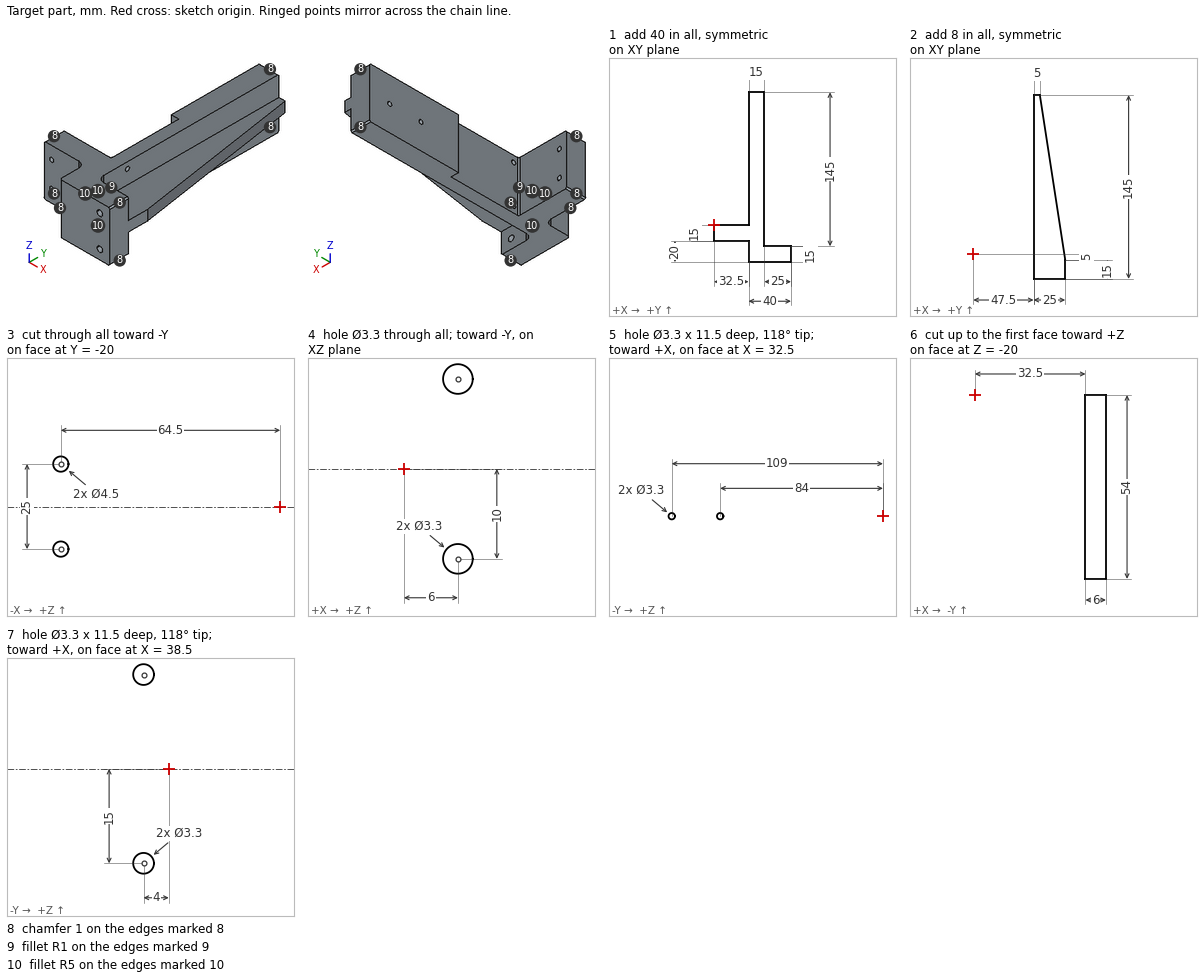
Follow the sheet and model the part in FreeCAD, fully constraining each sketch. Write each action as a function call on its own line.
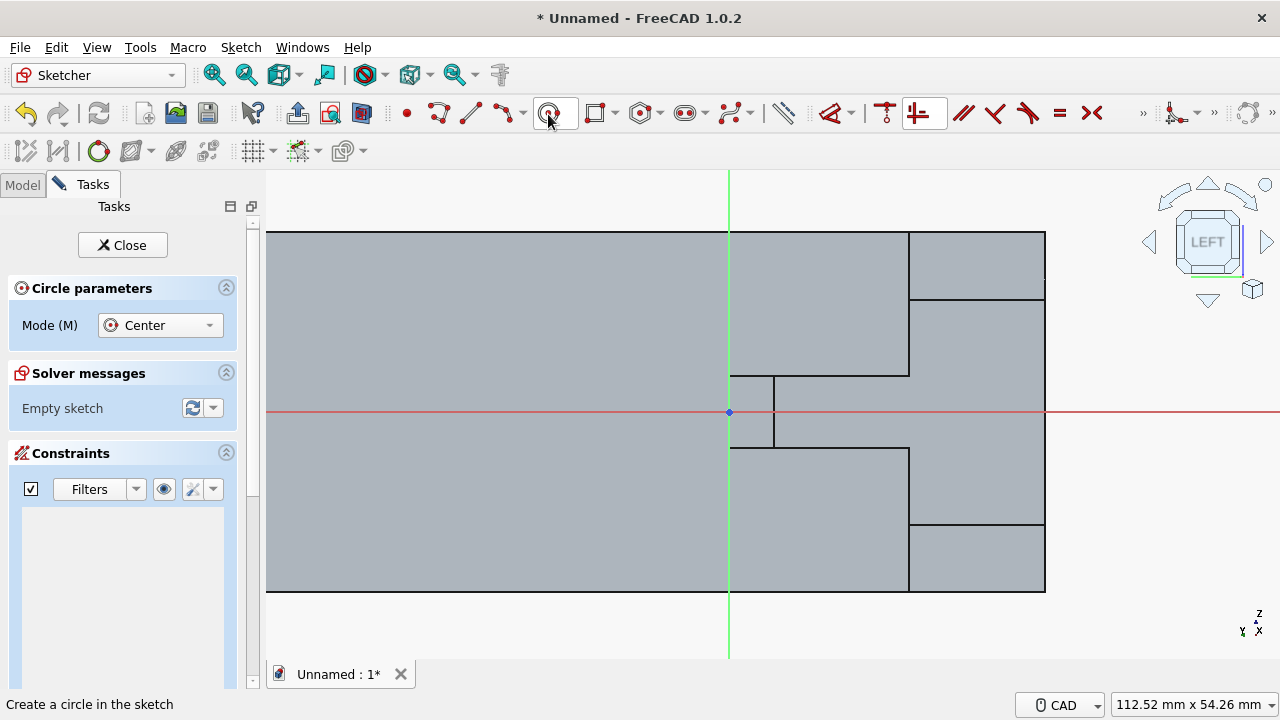
scroll(693, 547, up, 3)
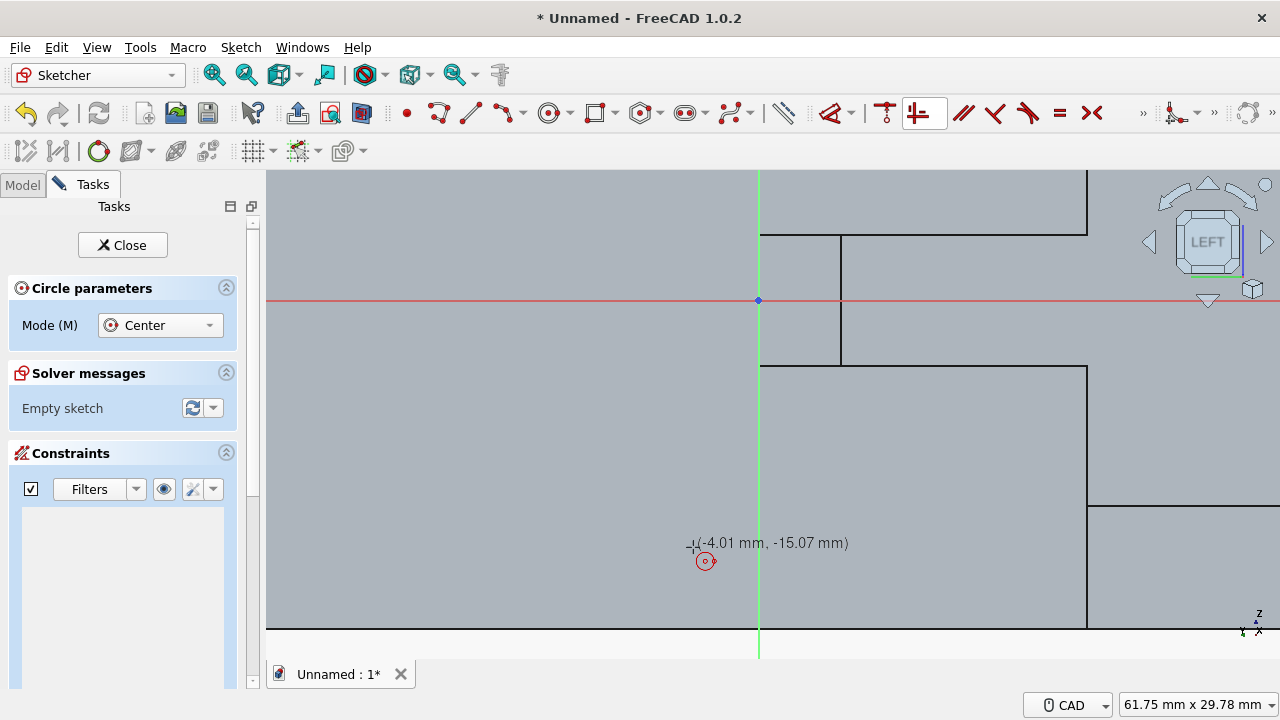
click(693, 547)
click(712, 528)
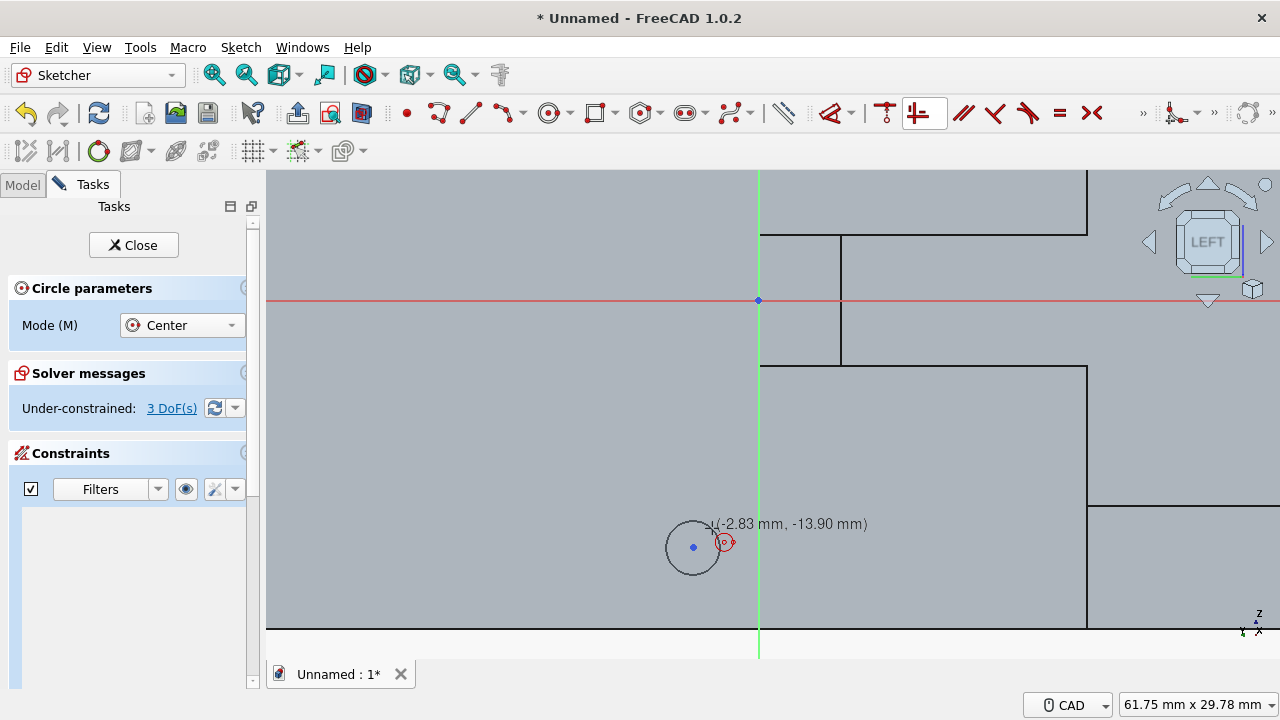
scroll(695, 553, down, 3)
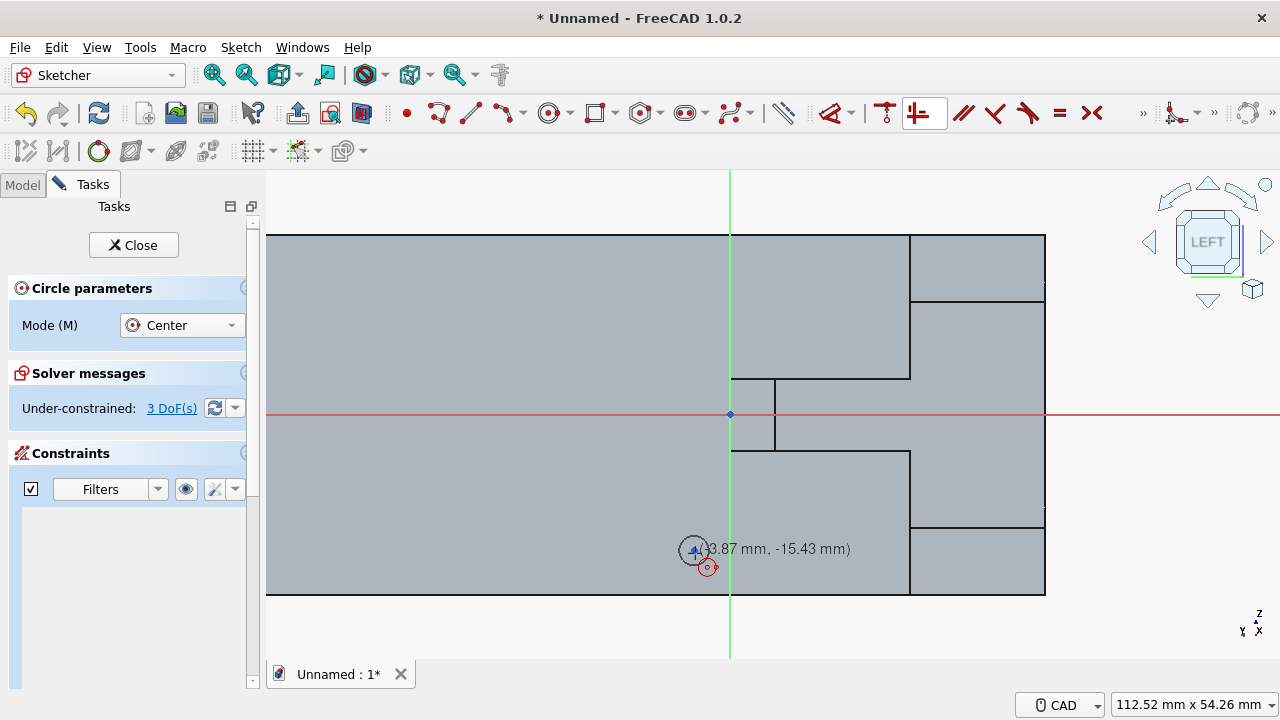
scroll(694, 280, up, 3)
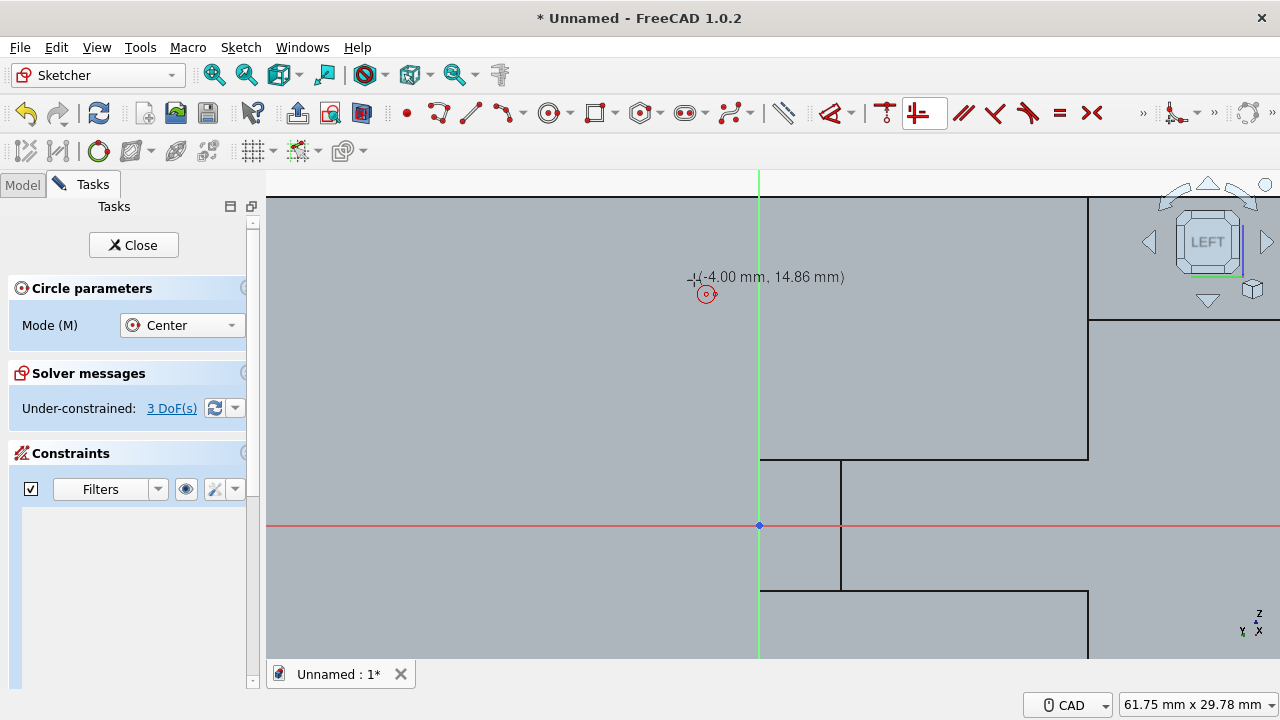
click(694, 279)
click(713, 260)
key(Escape)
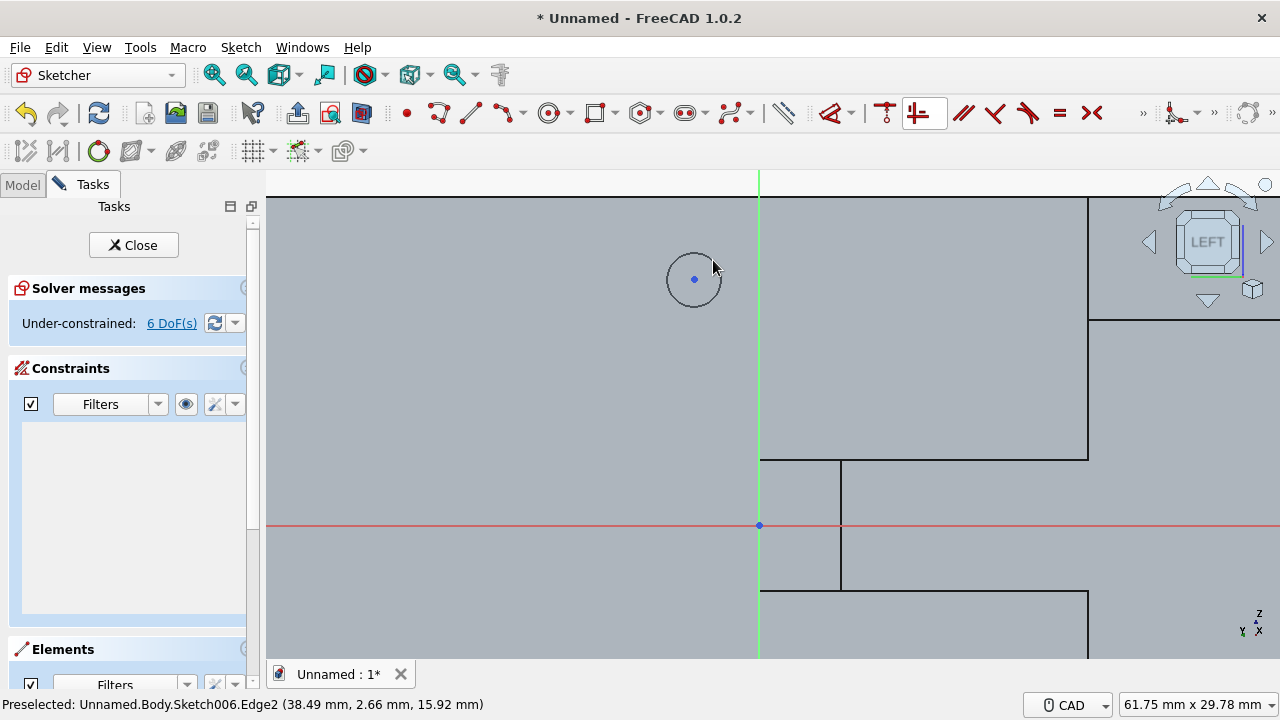
scroll(694, 279, down, 3)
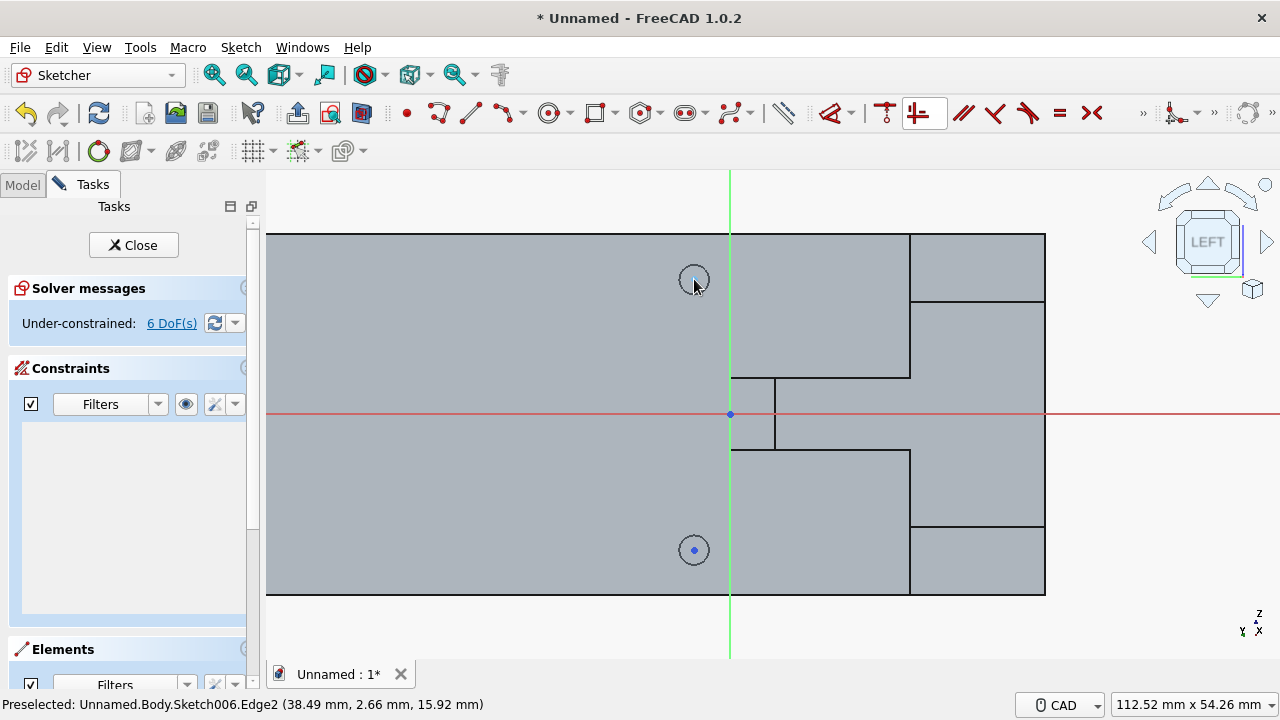
click(704, 540)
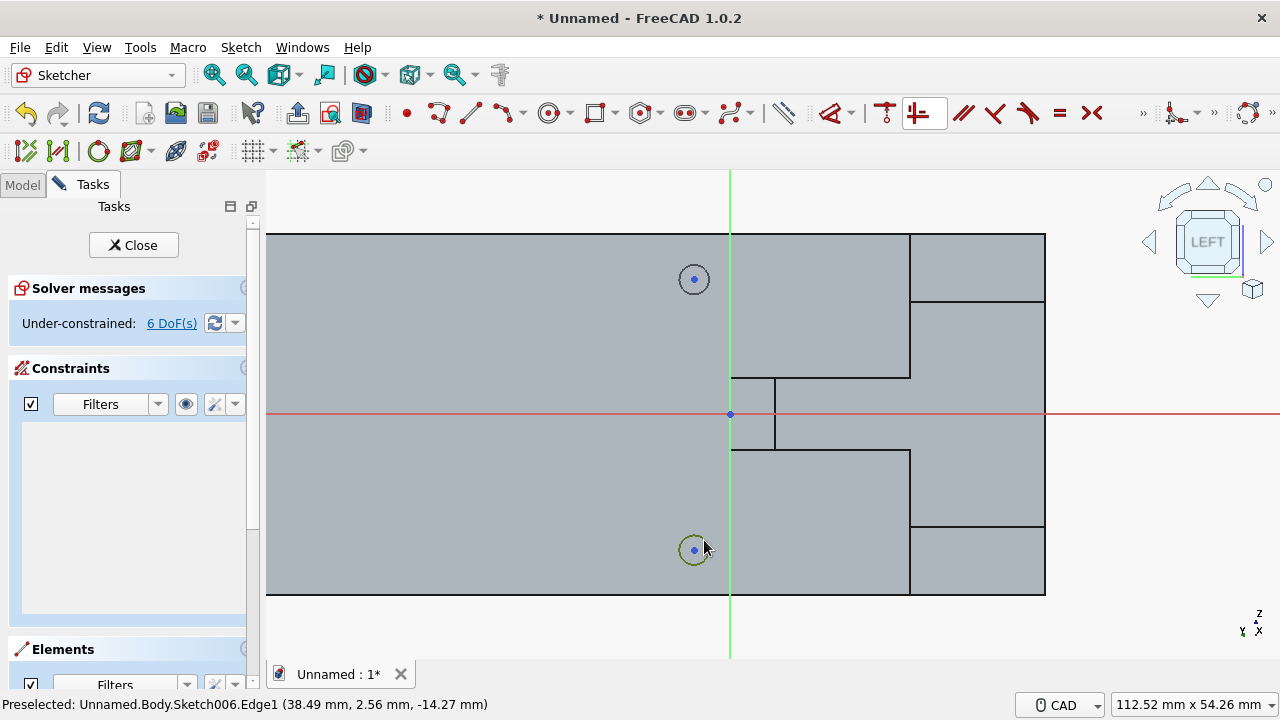
click(705, 269)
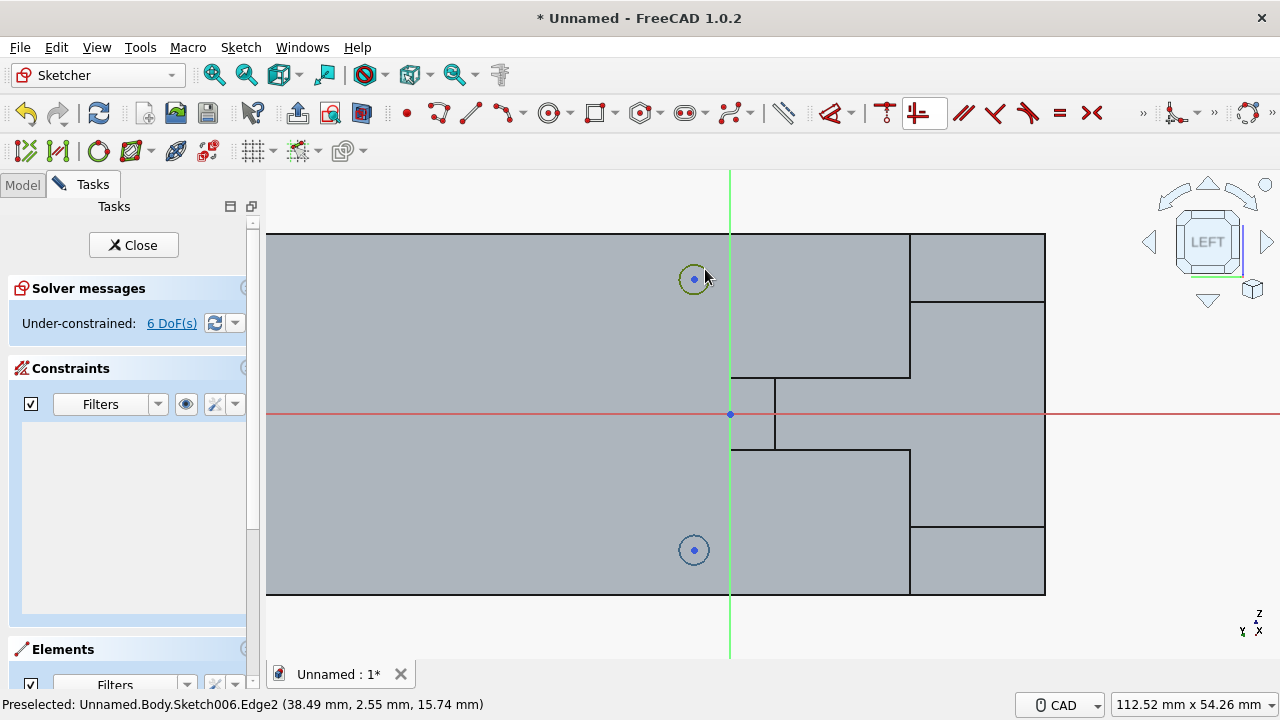
click(1060, 114)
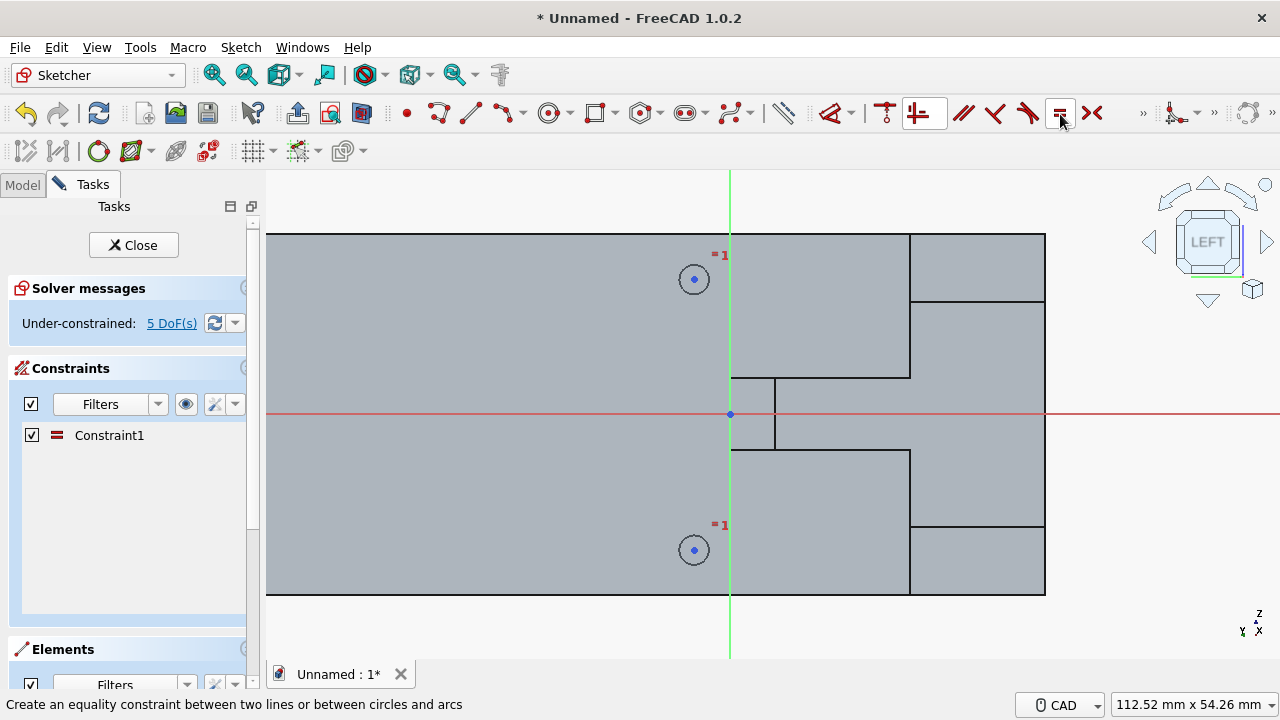
click(694, 550)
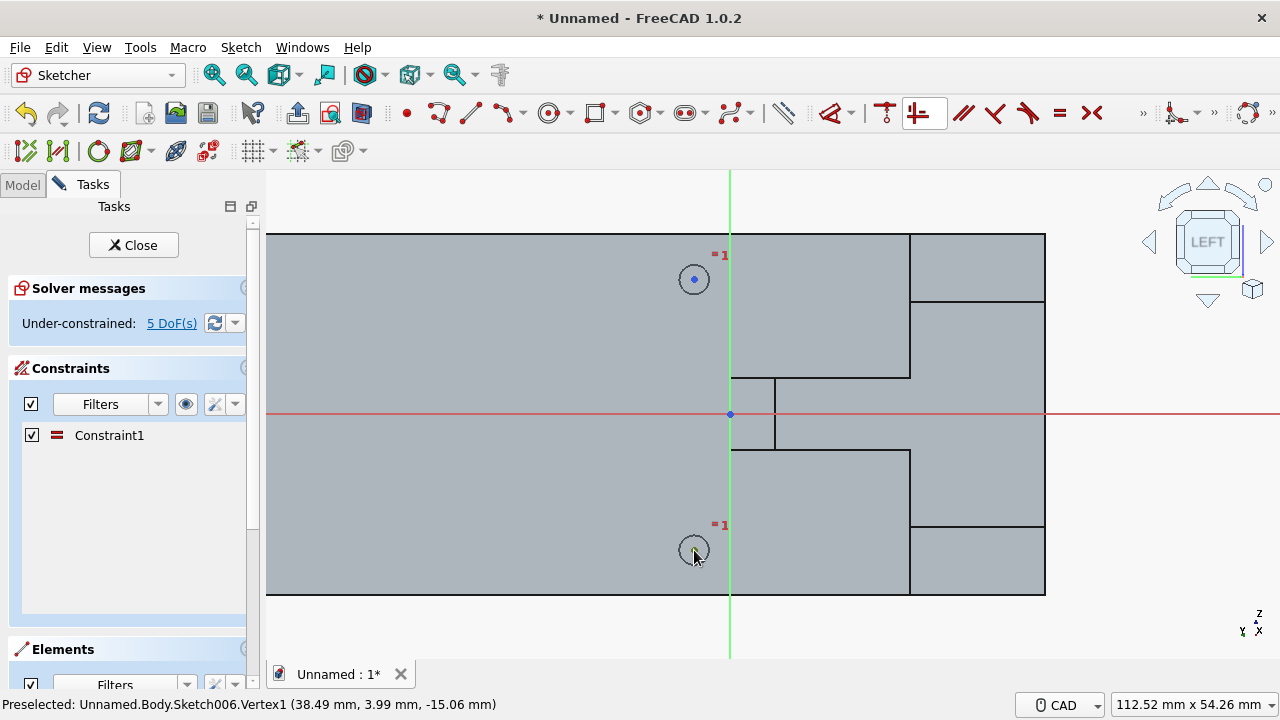
click(694, 280)